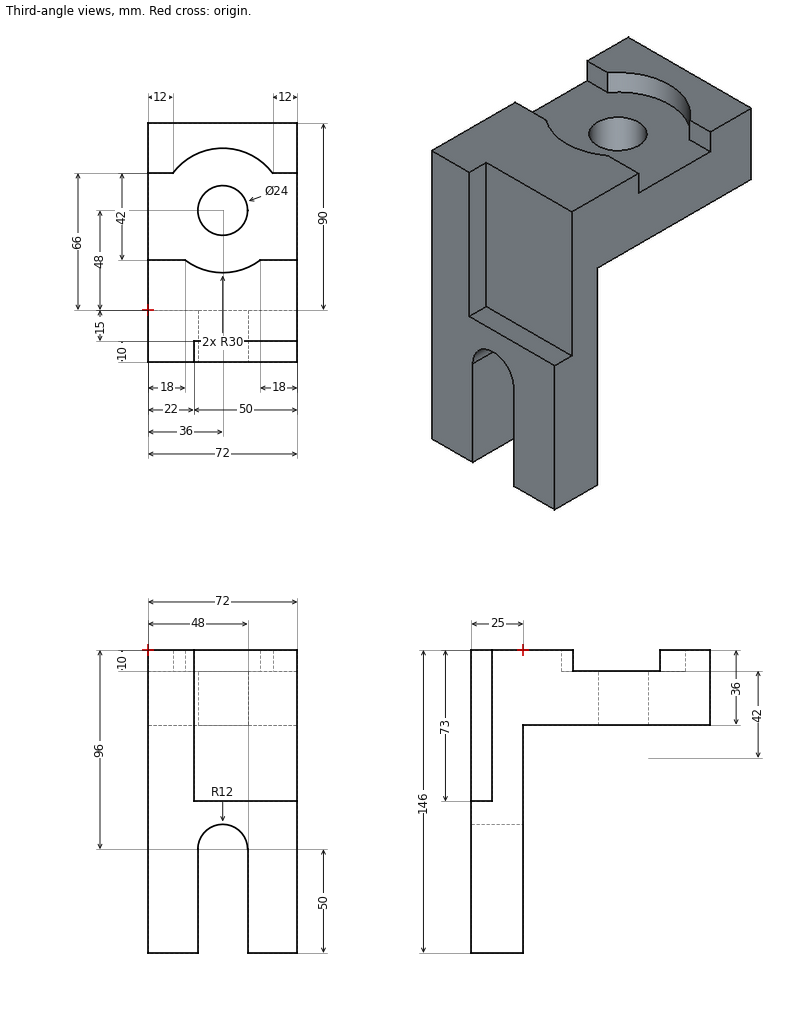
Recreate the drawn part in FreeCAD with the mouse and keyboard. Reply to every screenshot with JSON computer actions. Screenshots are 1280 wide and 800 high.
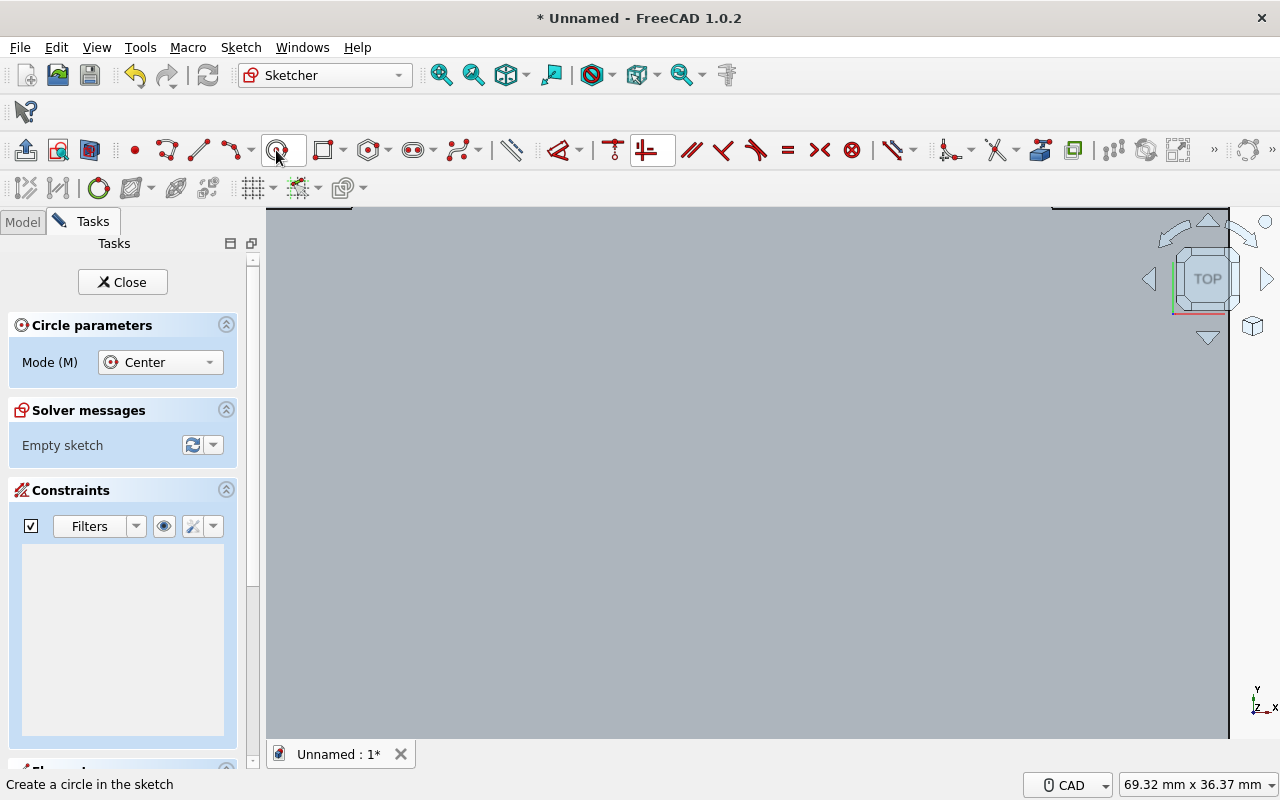
{"action": "left_click", "coordinate": [702, 472]}
{"action": "left_click", "coordinate": [826, 348]}
{"action": "key", "text": "Escape"}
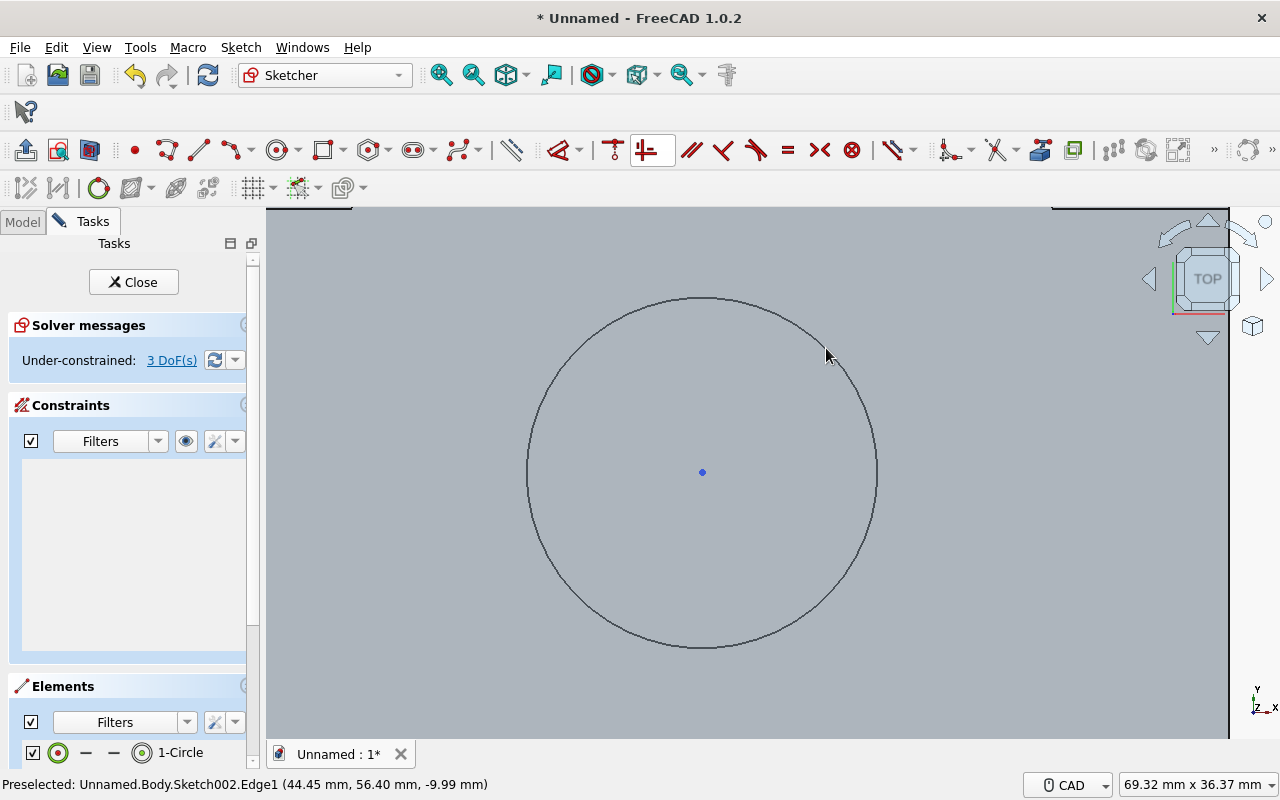
{"action": "key", "text": "d"}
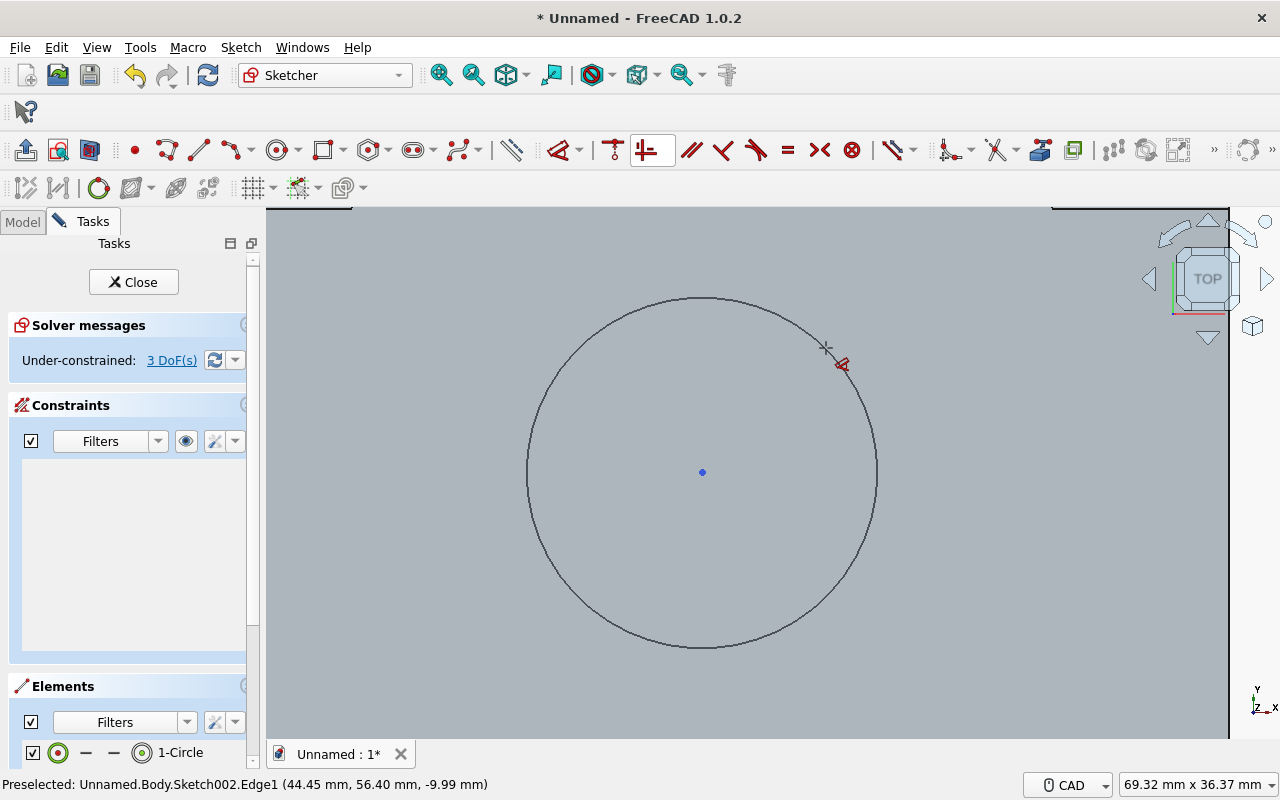
{"action": "left_click", "coordinate": [826, 349]}
{"action": "left_click", "coordinate": [849, 326]}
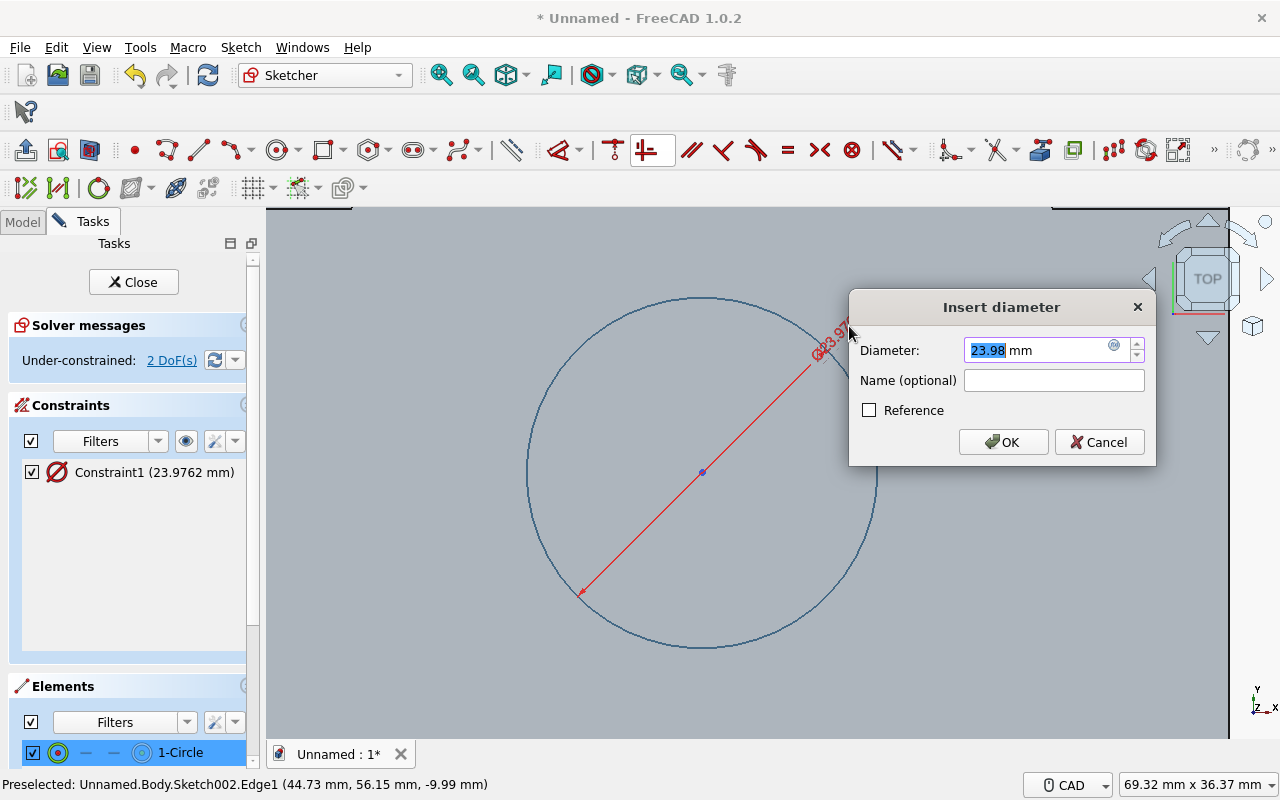
{"action": "type", "text": "24"}
{"action": "key", "text": "Return"}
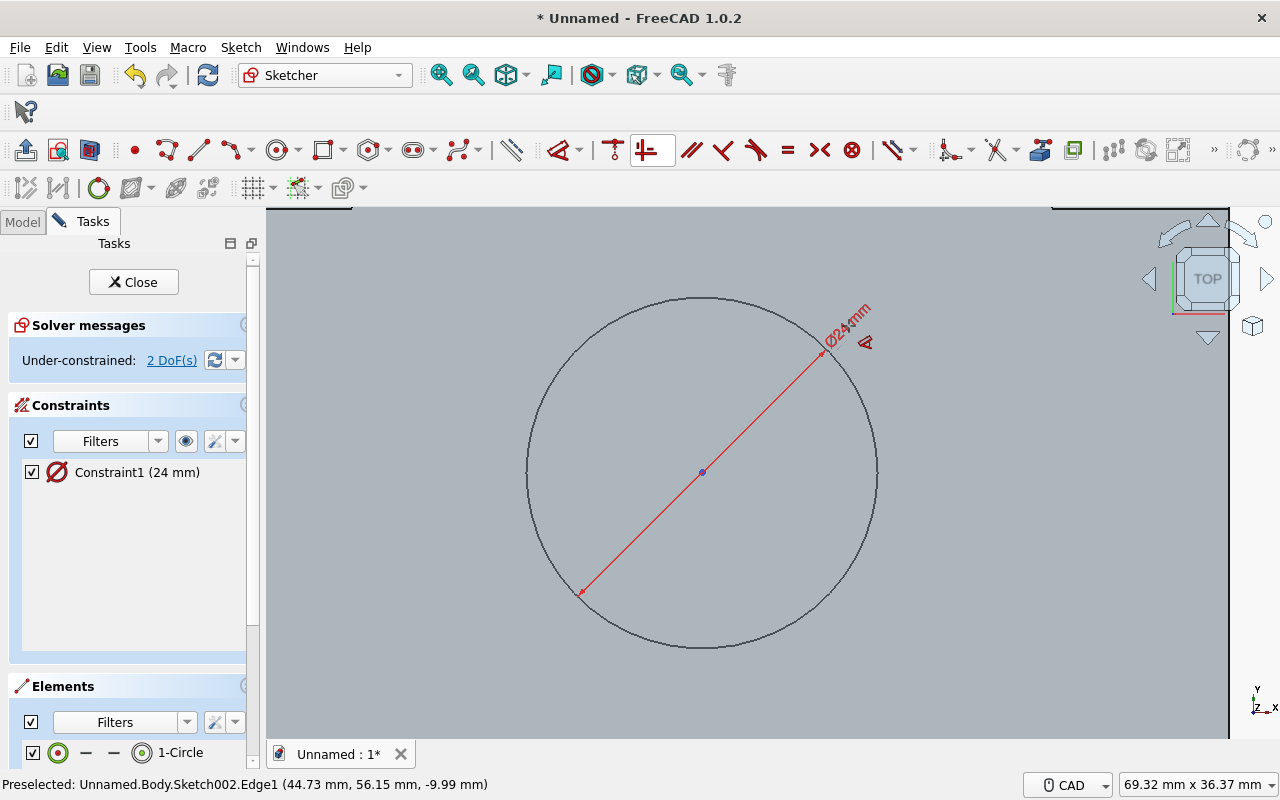
{"action": "left_click", "coordinate": [702, 473]}
{"action": "left_click", "coordinate": [498, 439]}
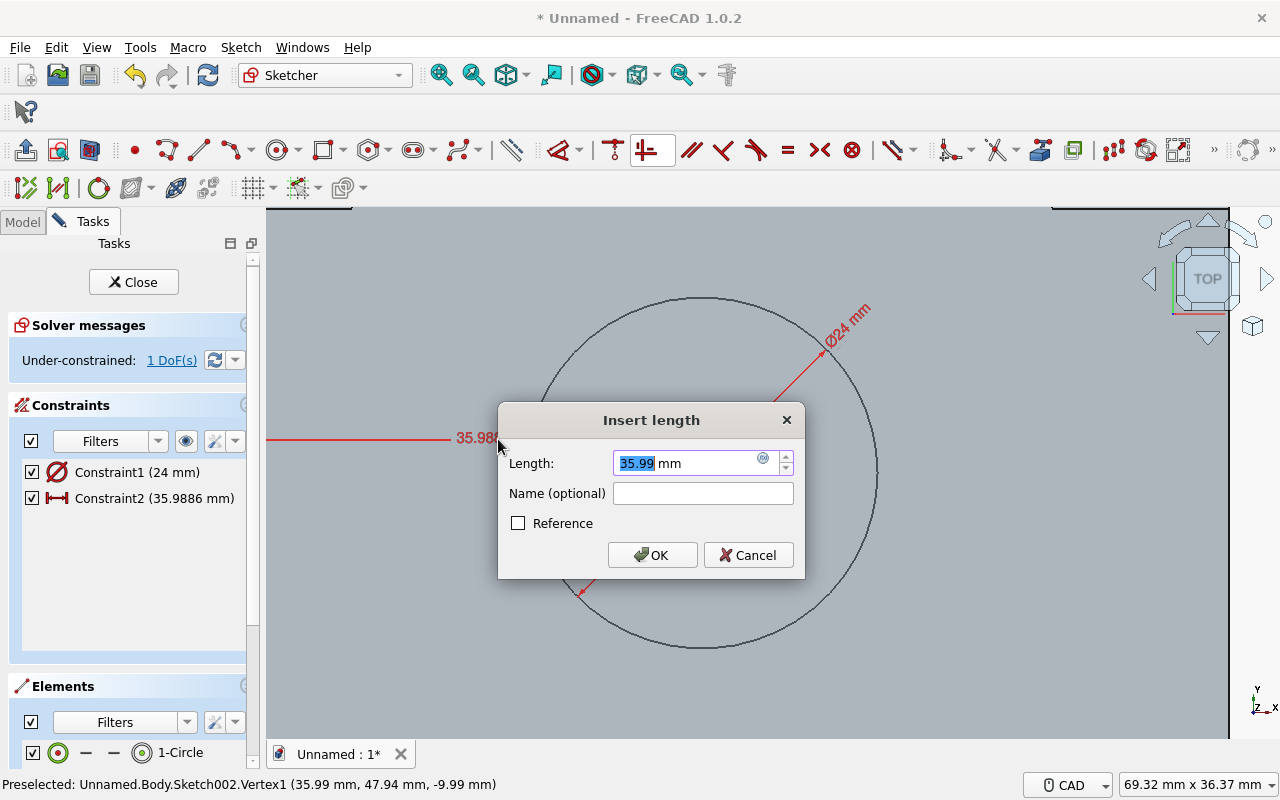
{"action": "type", "text": "36"}
{"action": "key", "text": "Return"}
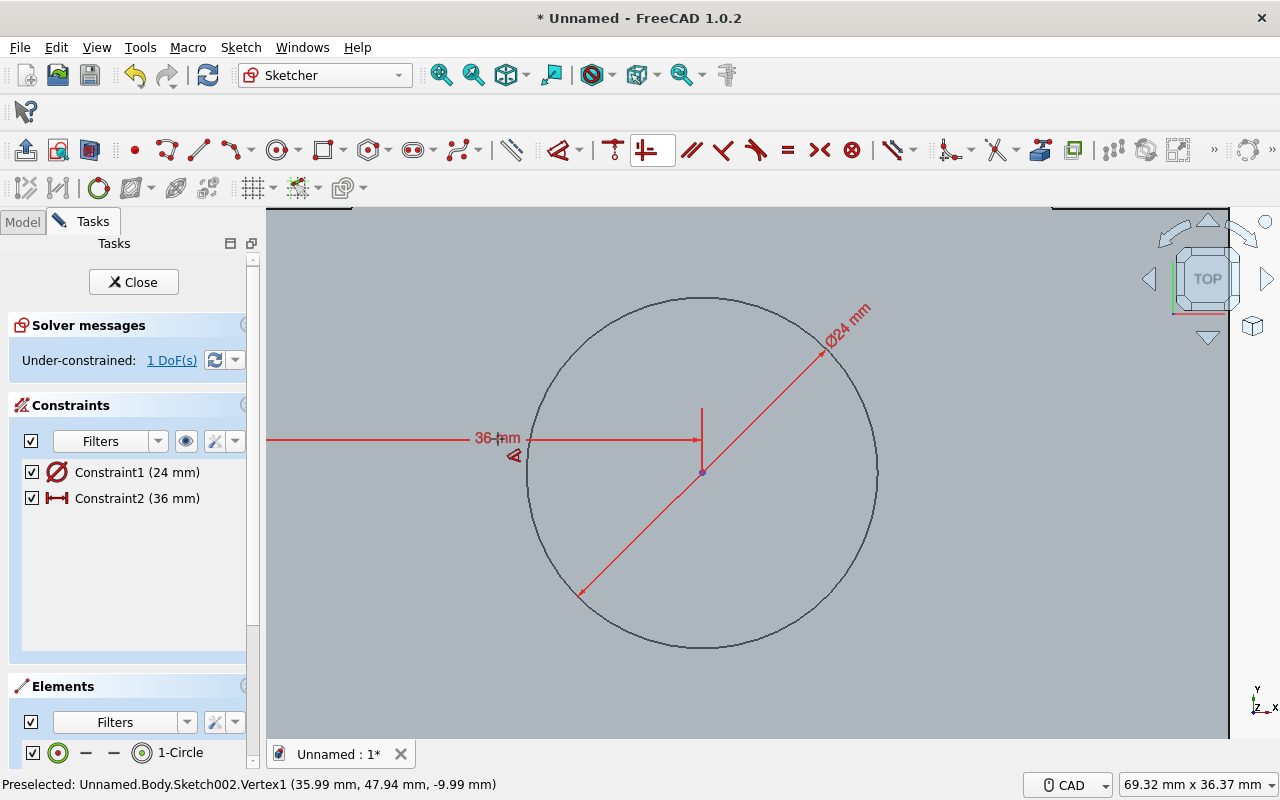
{"action": "left_click", "coordinate": [702, 473]}
{"action": "left_click", "coordinate": [736, 592]}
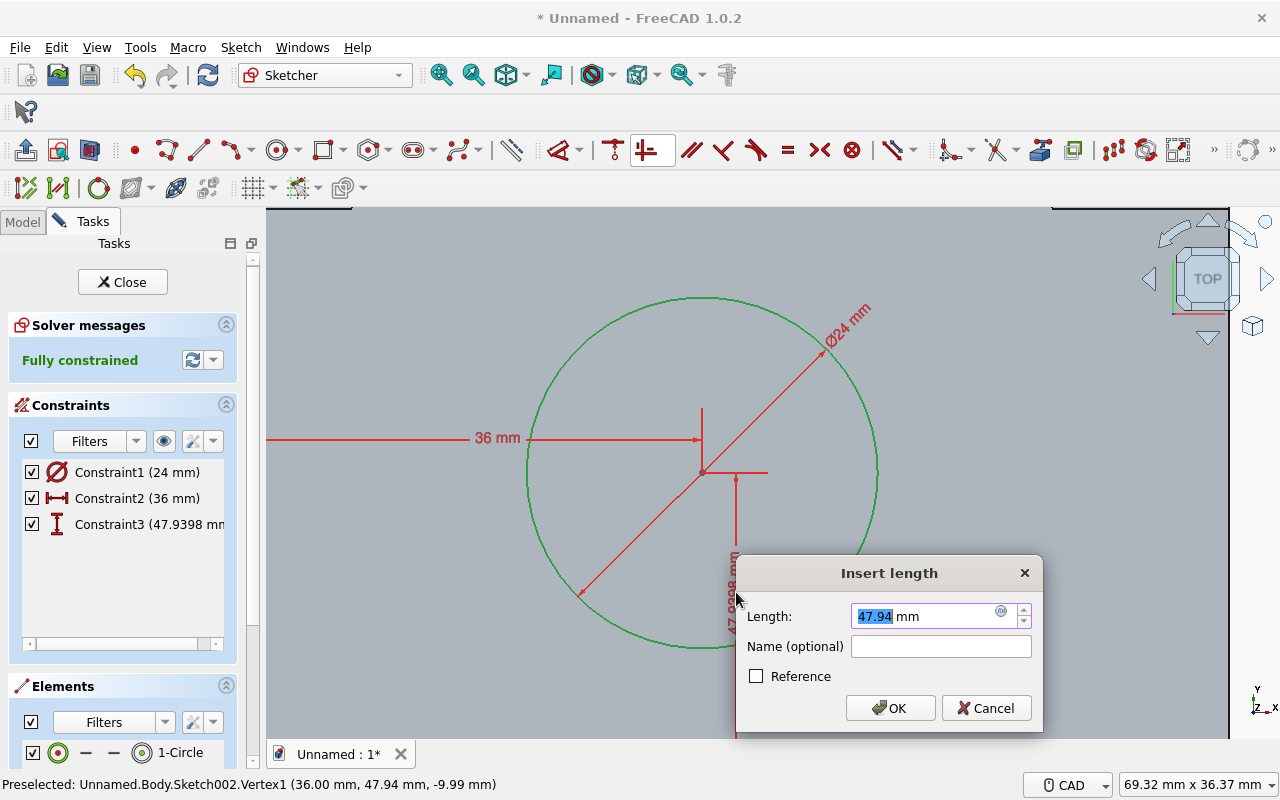
{"action": "type", "text": "48"}
{"action": "key", "text": "Return"}
{"action": "key", "text": "Escape"}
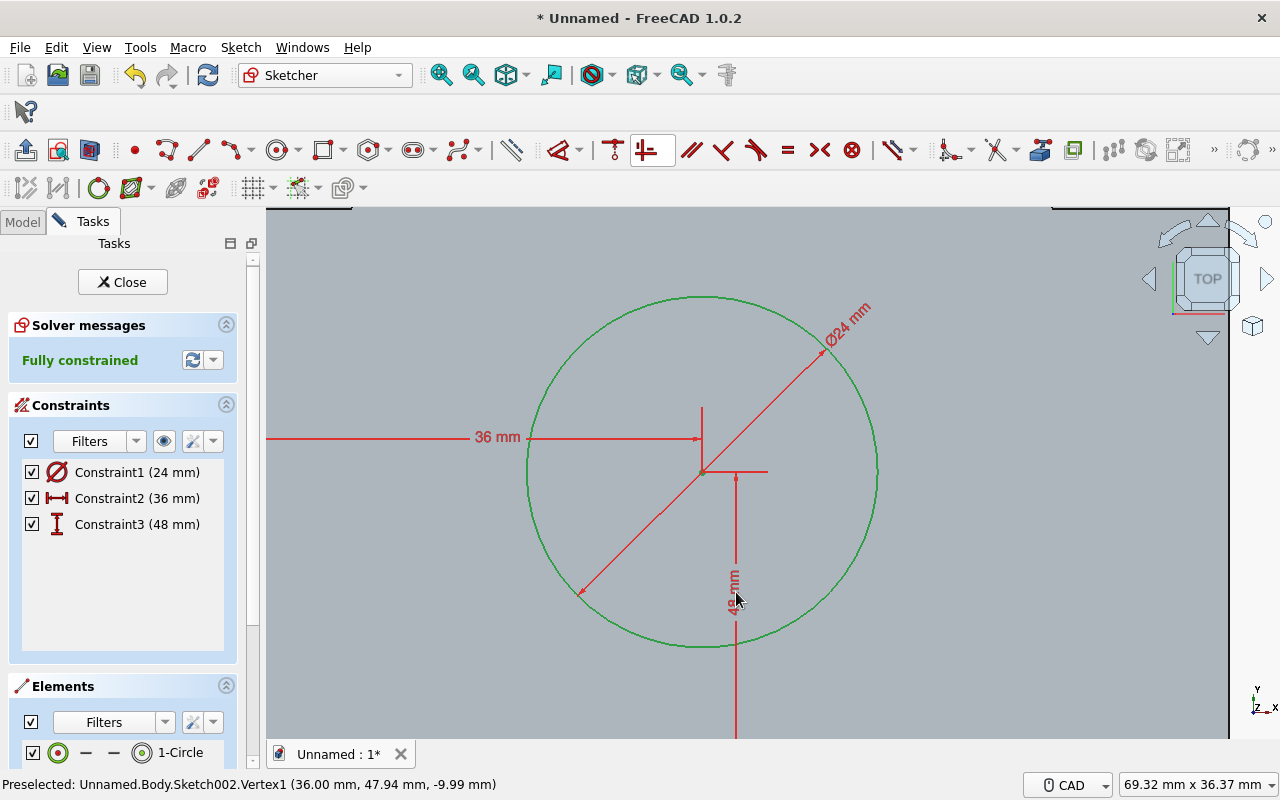
{"action": "left_click", "coordinate": [123, 282]}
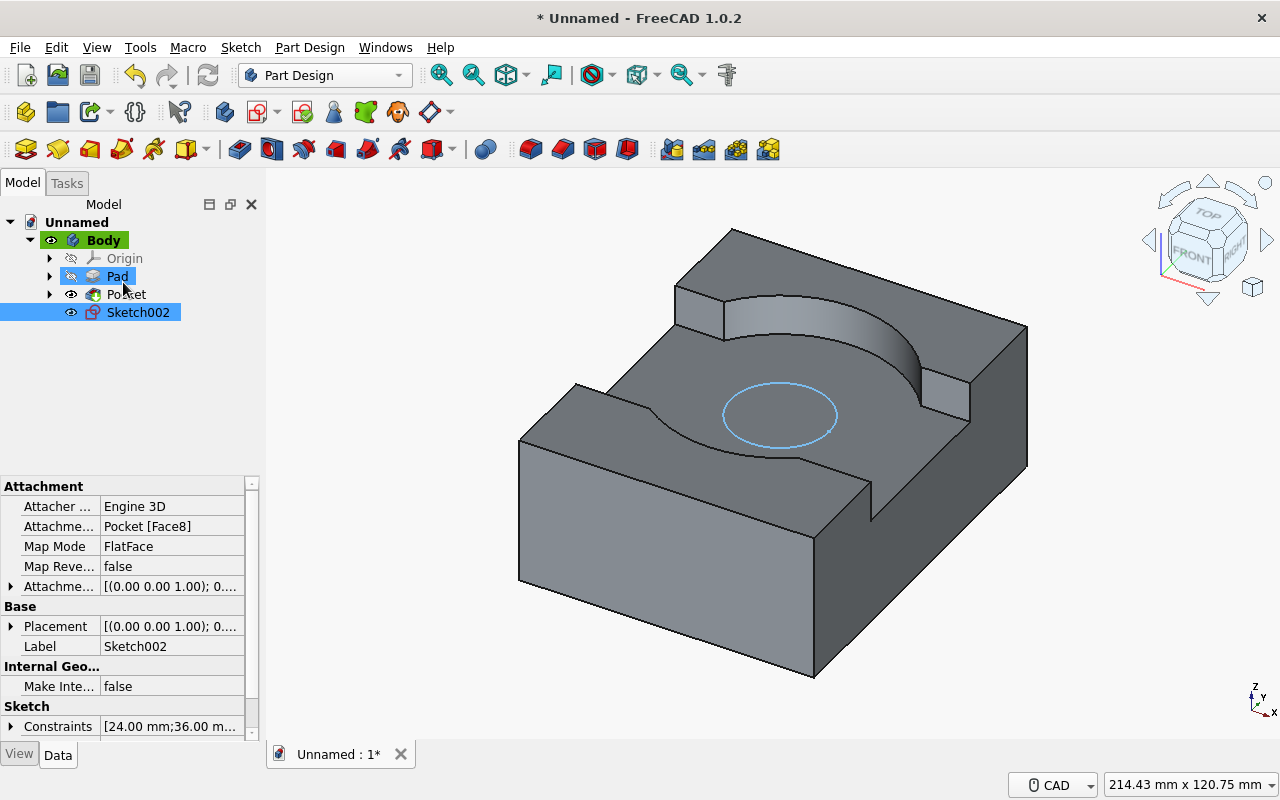
{"action": "left_click", "coordinate": [240, 150]}